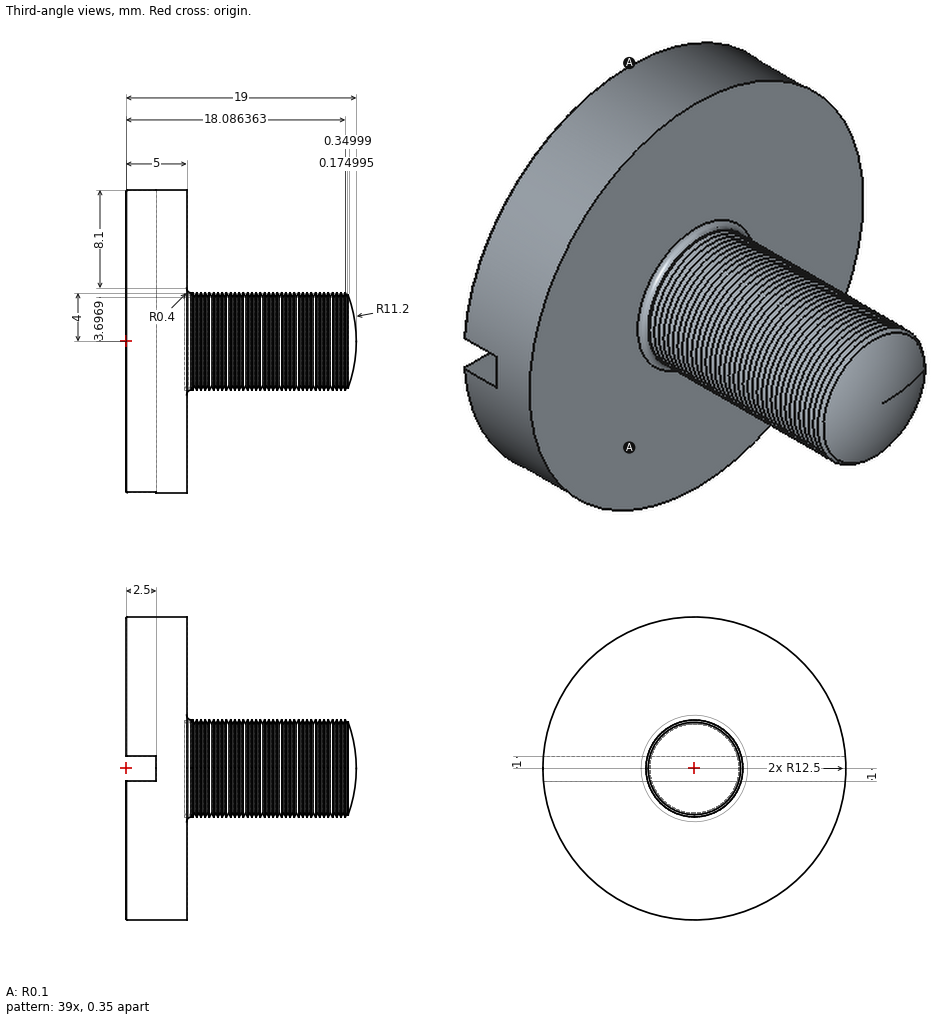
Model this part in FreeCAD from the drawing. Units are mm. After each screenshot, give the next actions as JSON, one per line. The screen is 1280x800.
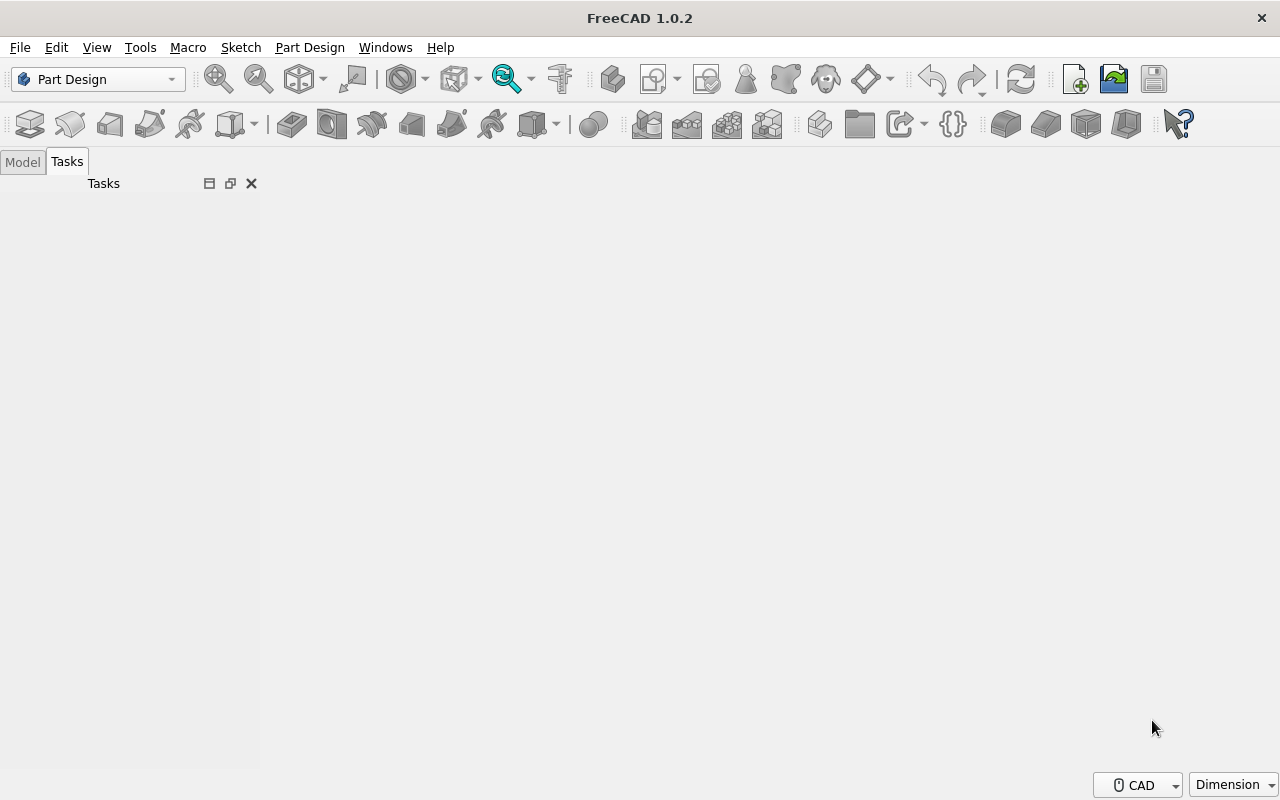
{"action": "left_click", "coordinate": [1074, 80]}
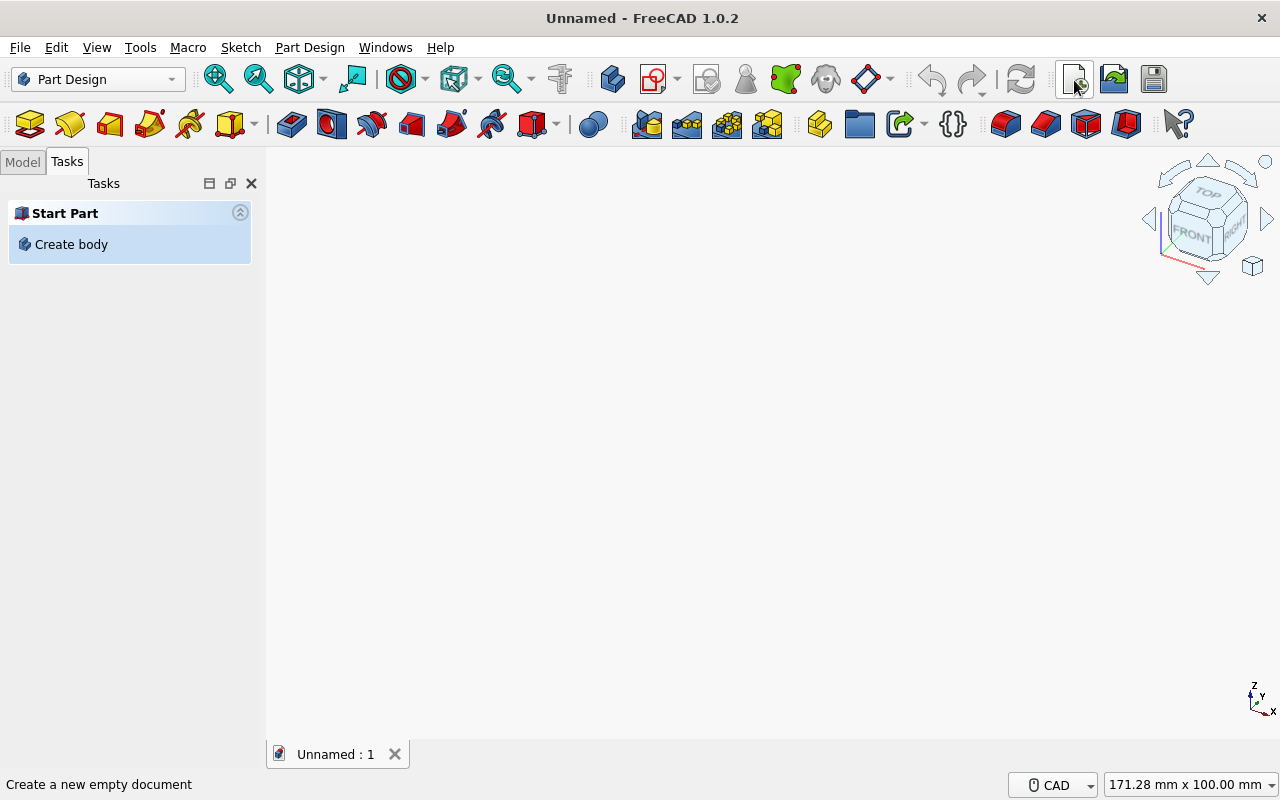
{"action": "left_click", "coordinate": [654, 80]}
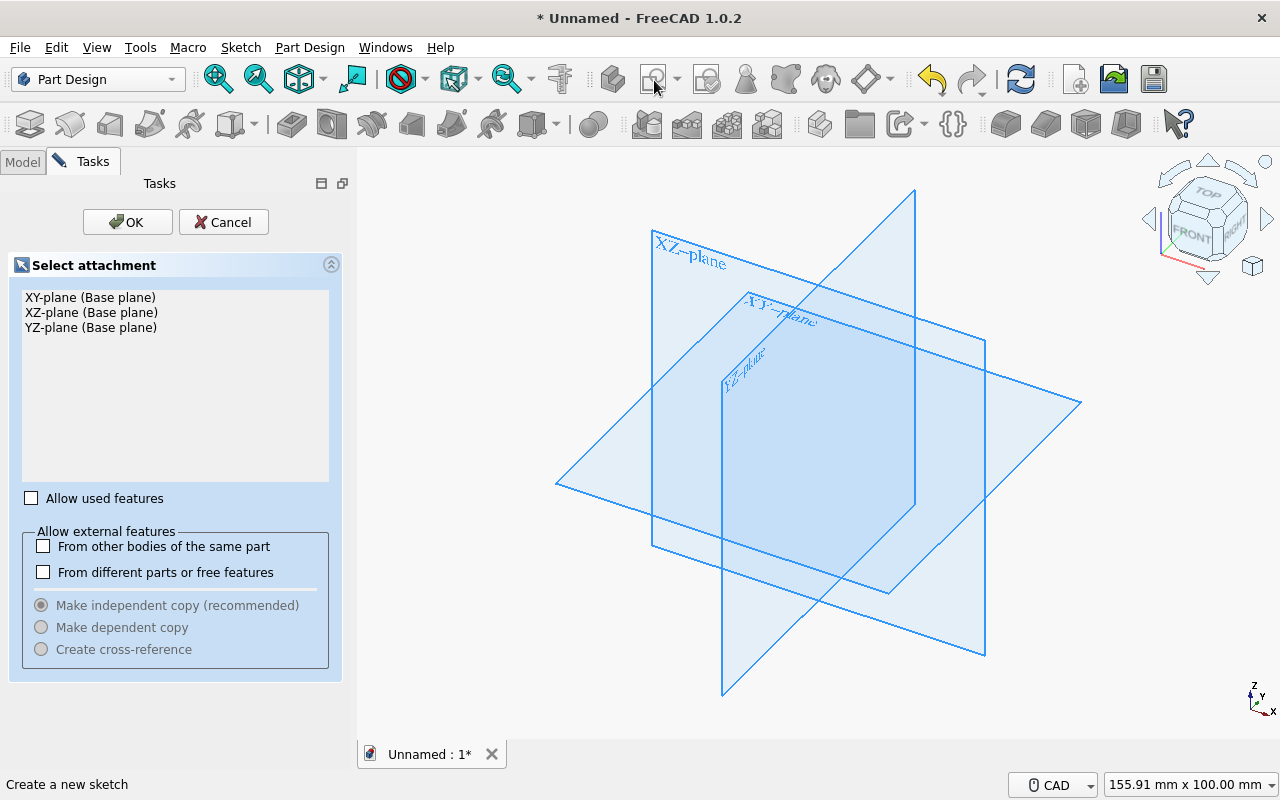
{"action": "left_click", "coordinate": [82, 298]}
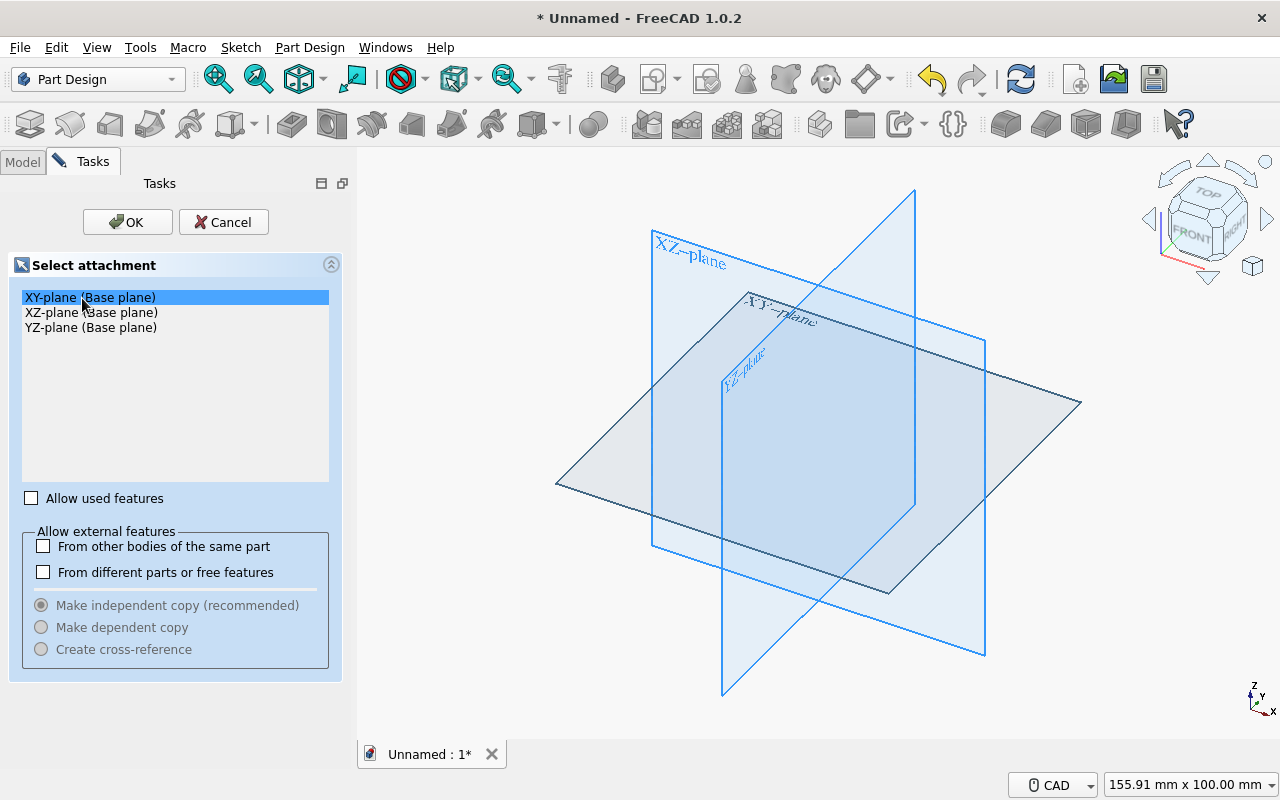
{"action": "left_click", "coordinate": [128, 222]}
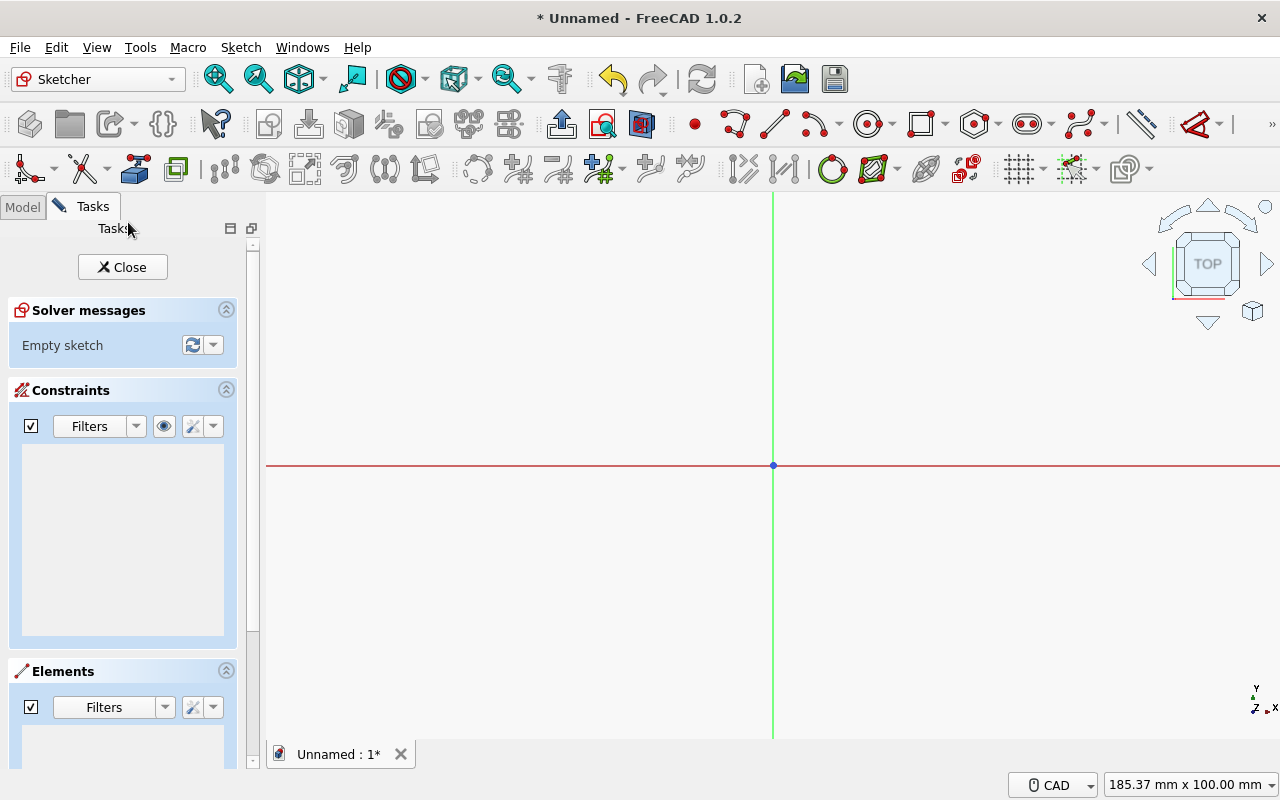
{"action": "scroll", "coordinate": [855, 423], "scroll_direction": "up", "scroll_amount": 8}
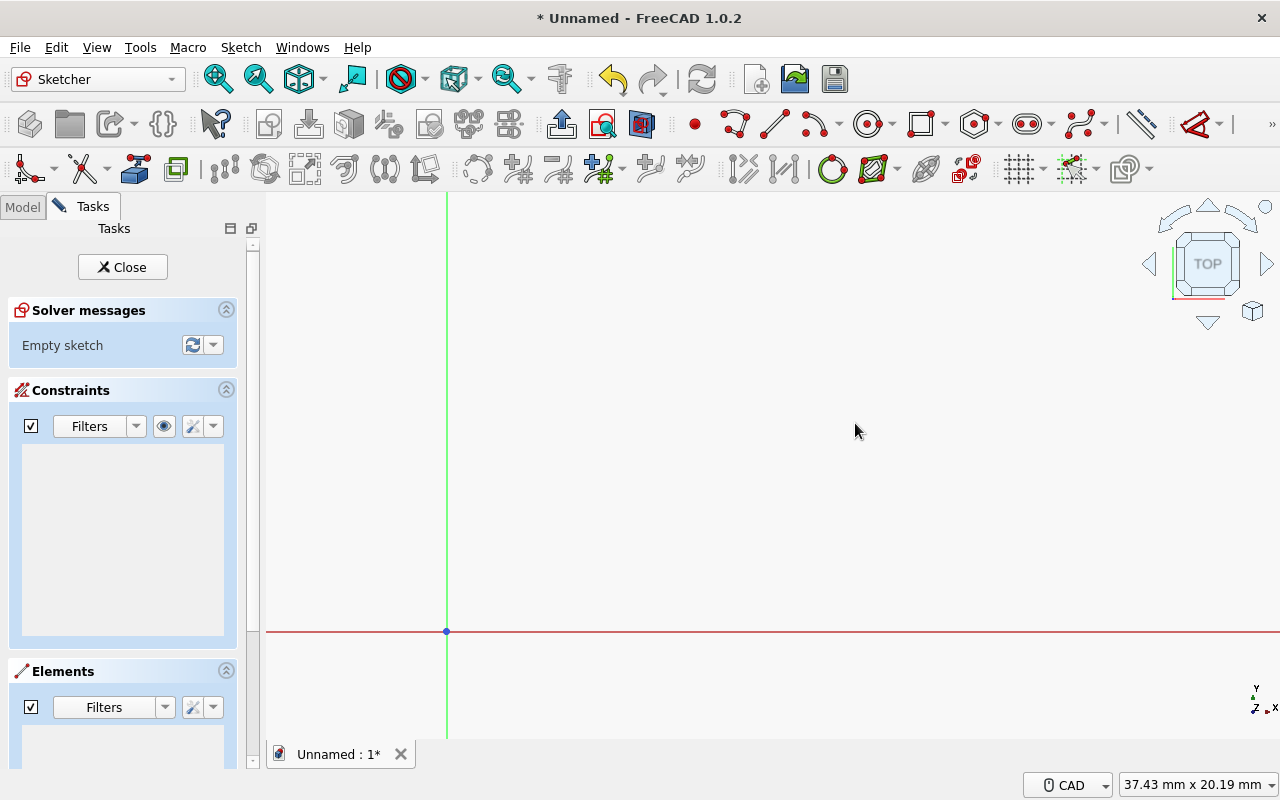
{"action": "left_click", "coordinate": [776, 124]}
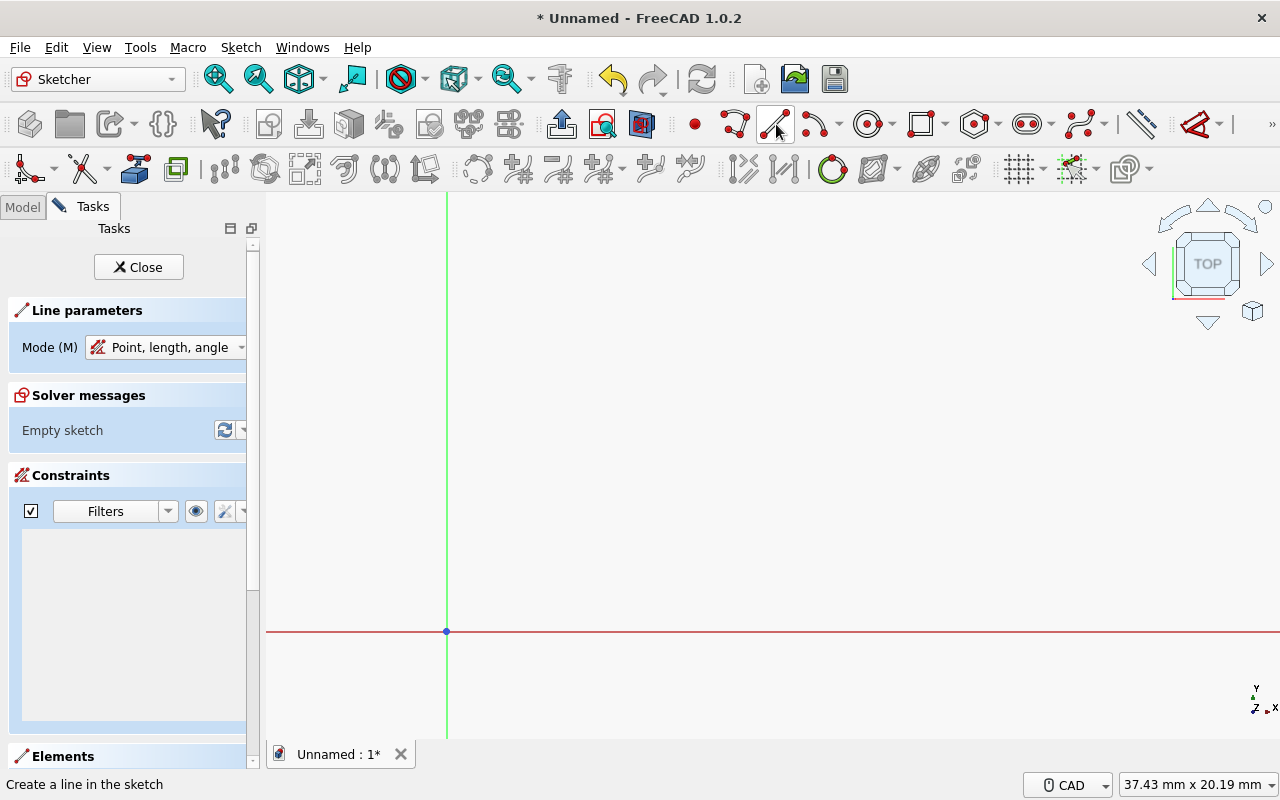
{"action": "left_click", "coordinate": [941, 523]}
{"action": "left_click", "coordinate": [593, 523]}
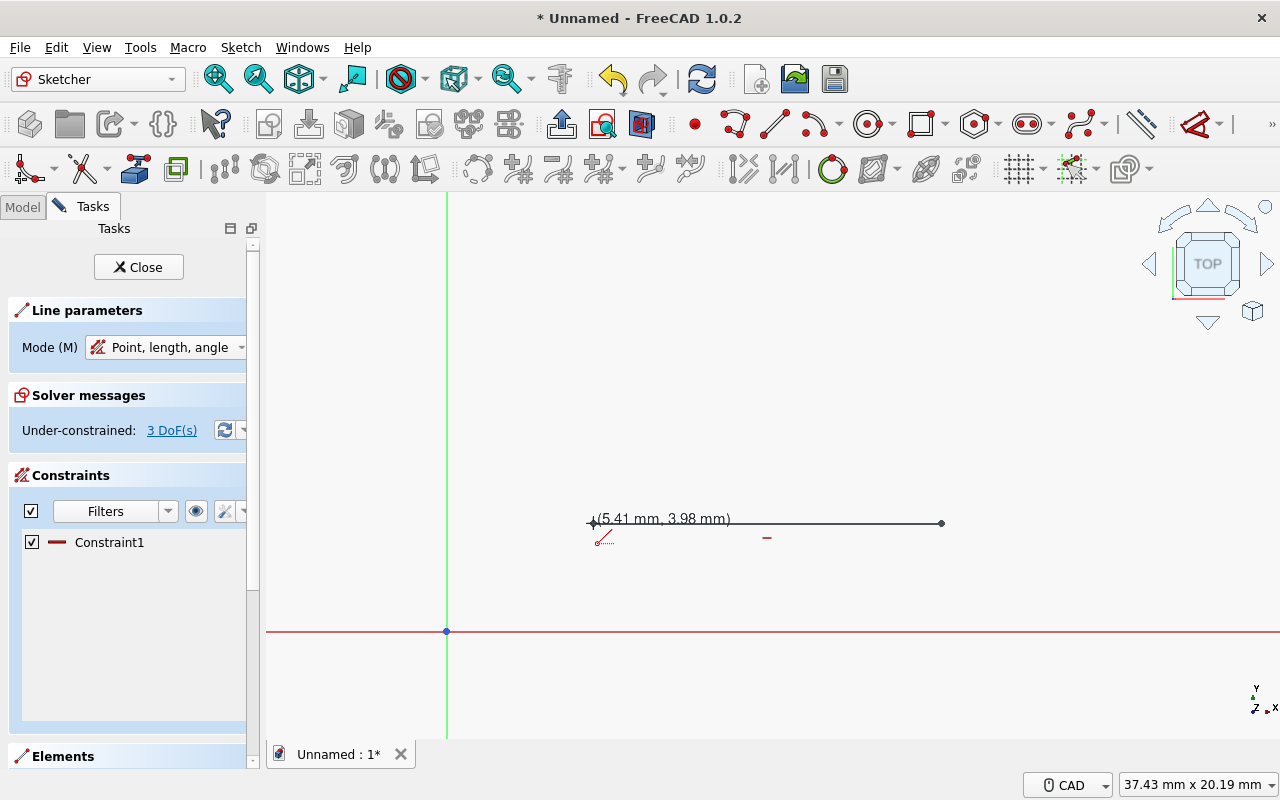
{"action": "left_click", "coordinate": [736, 124]}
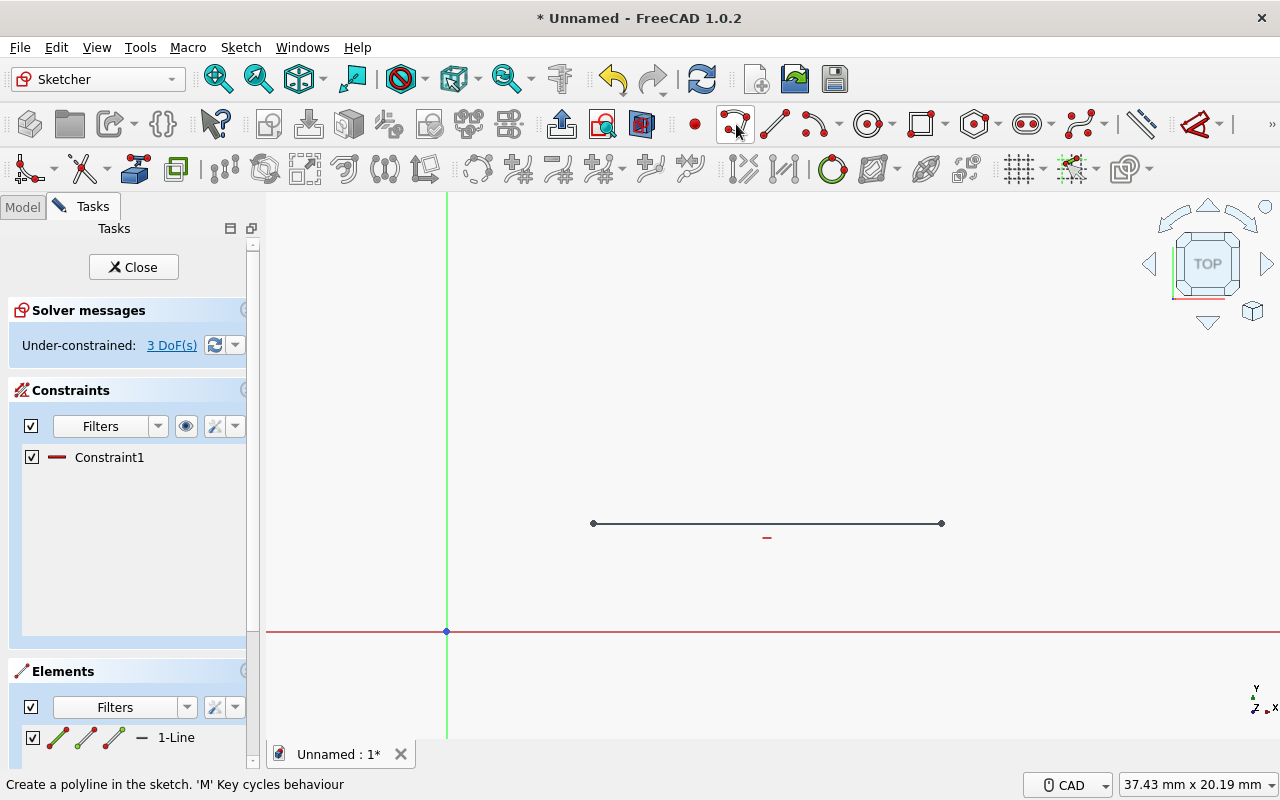
{"action": "left_click", "coordinate": [582, 513]}
{"action": "left_click", "coordinate": [582, 293]}
{"action": "left_click", "coordinate": [447, 293]}
{"action": "left_click", "coordinate": [447, 632]}
{"action": "left_click", "coordinate": [961, 623]}
{"action": "right_click", "coordinate": [961, 623]}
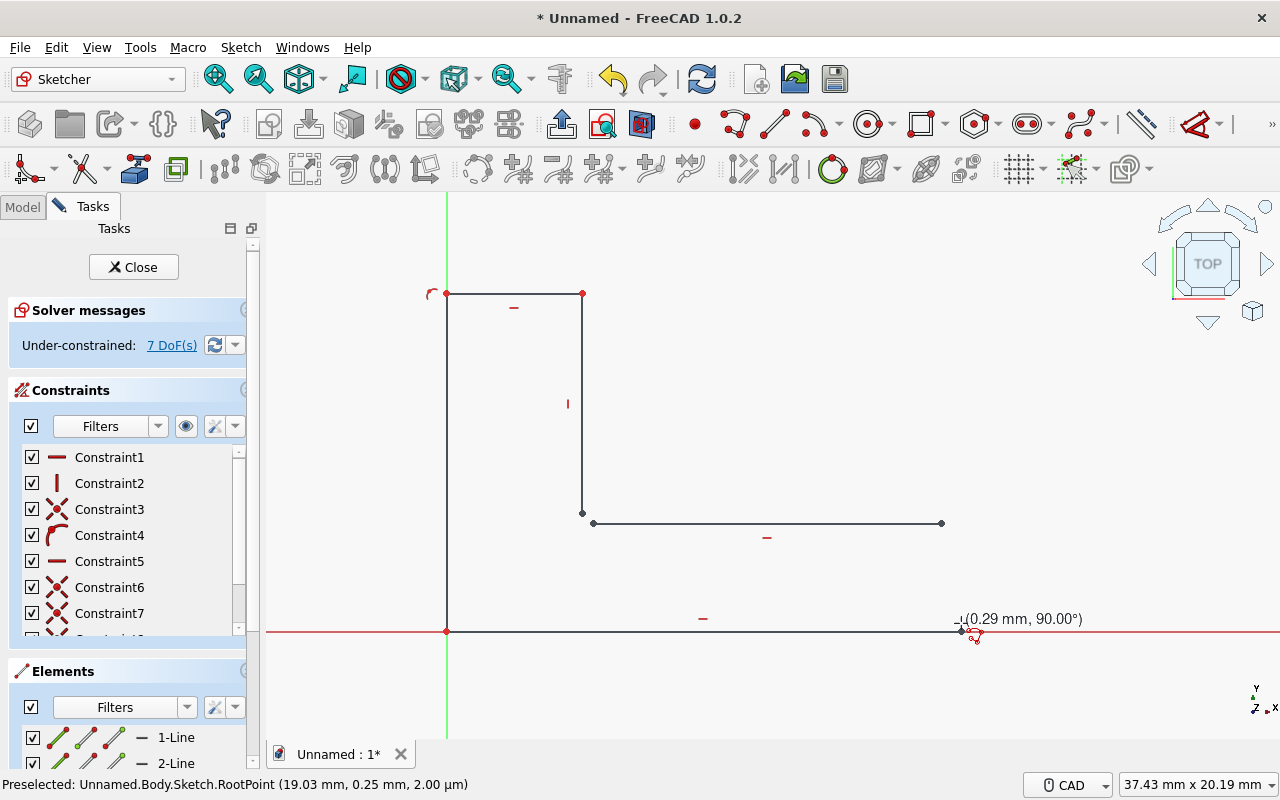
{"action": "left_click", "coordinate": [842, 124]}